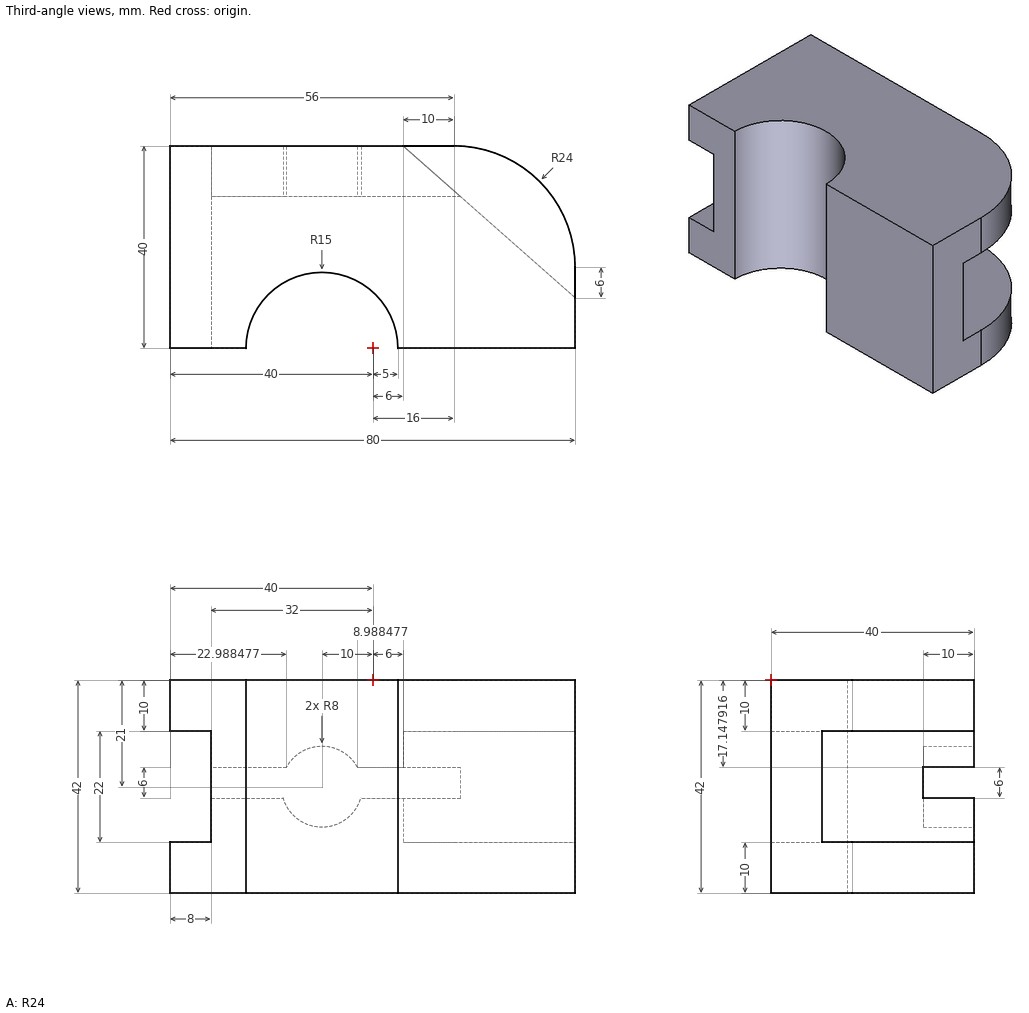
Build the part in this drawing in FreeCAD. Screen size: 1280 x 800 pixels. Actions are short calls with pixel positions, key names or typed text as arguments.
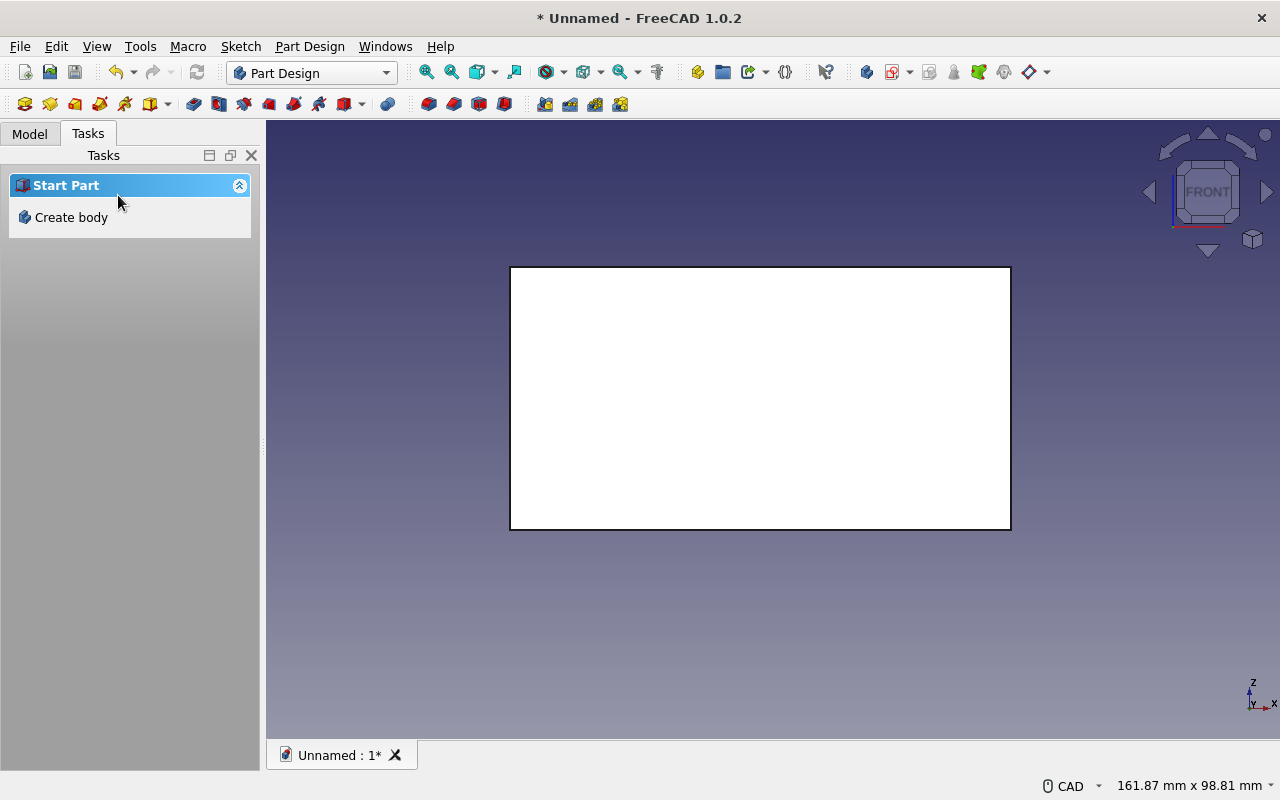
key(3)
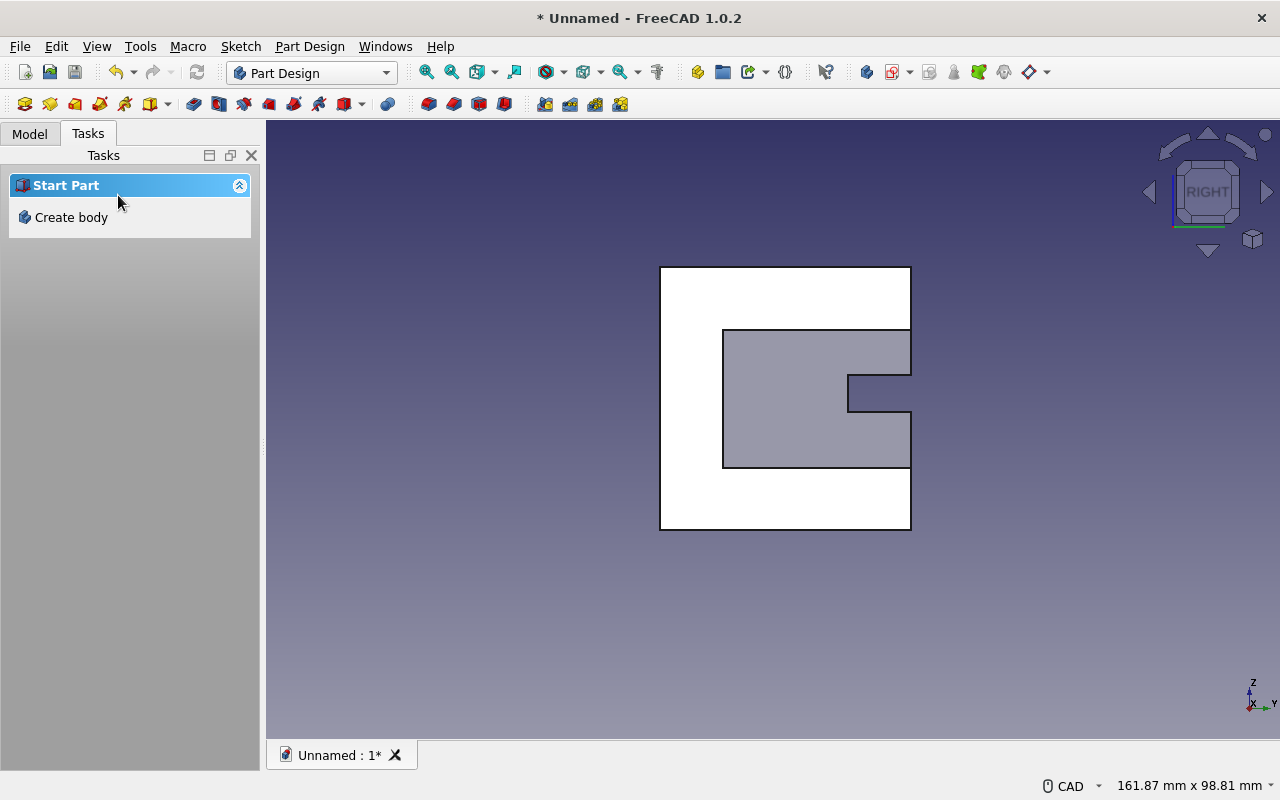
key(v)
key(f)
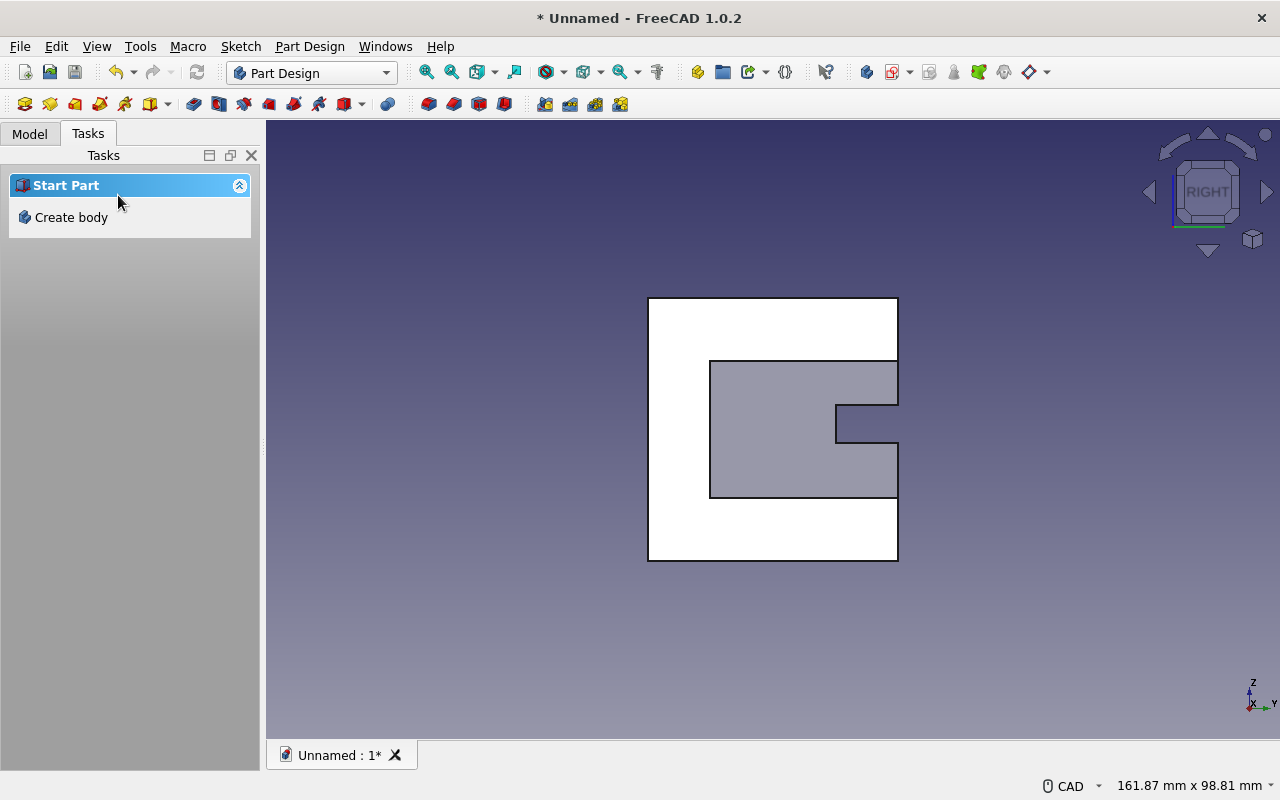
click(898, 529)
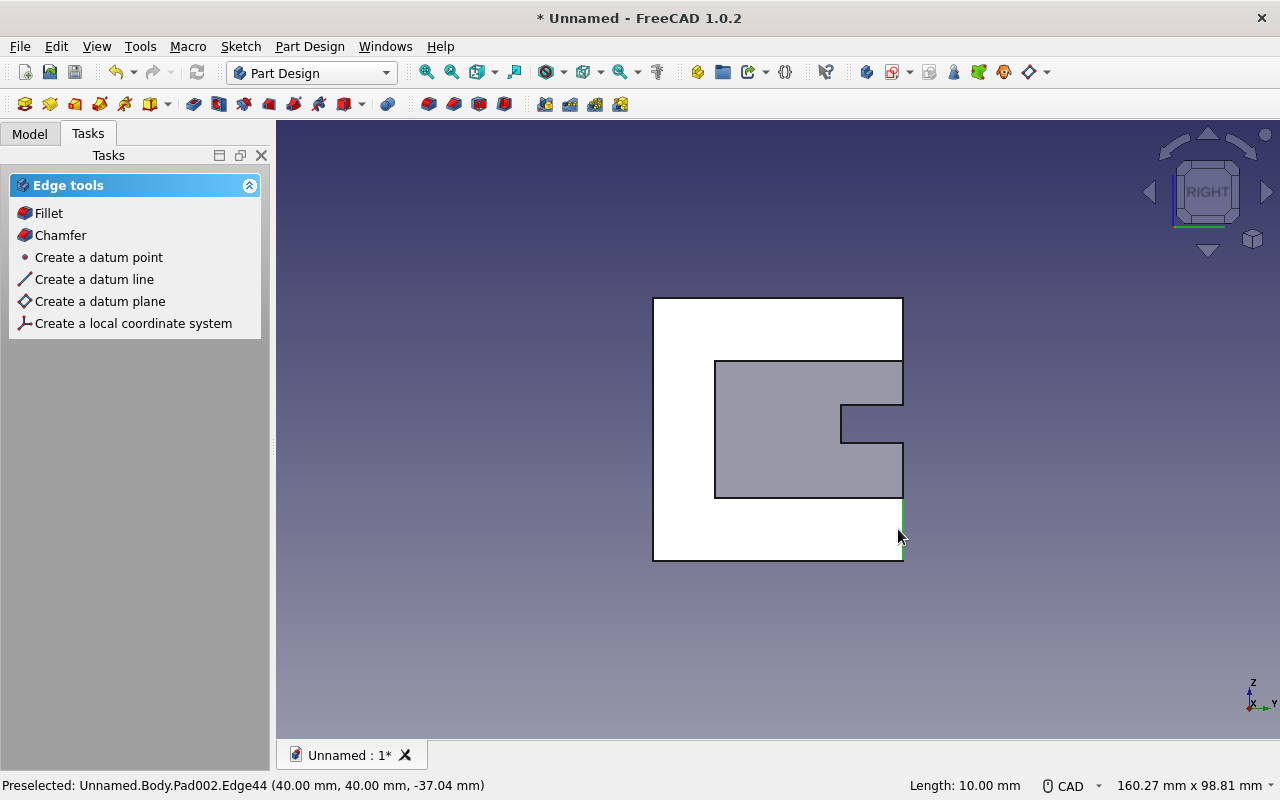
click(903, 328, ctrl)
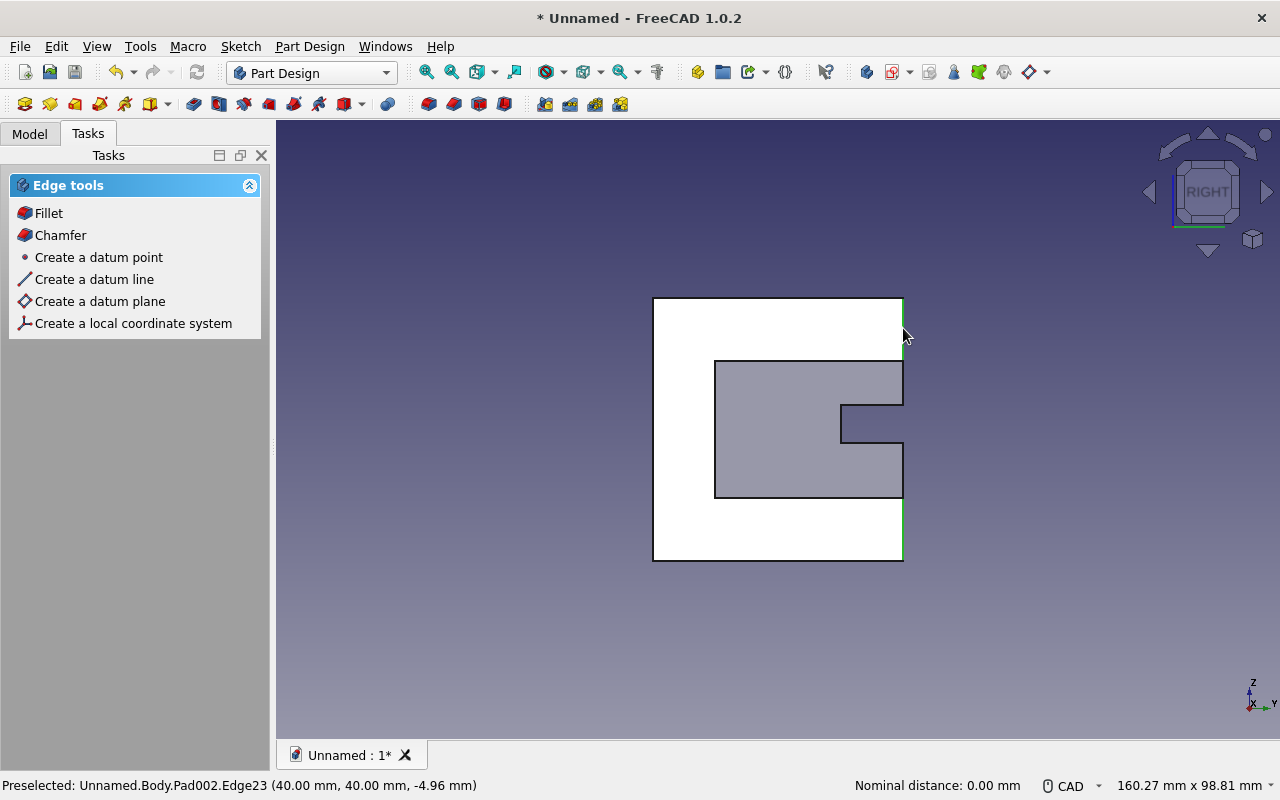
click(429, 104)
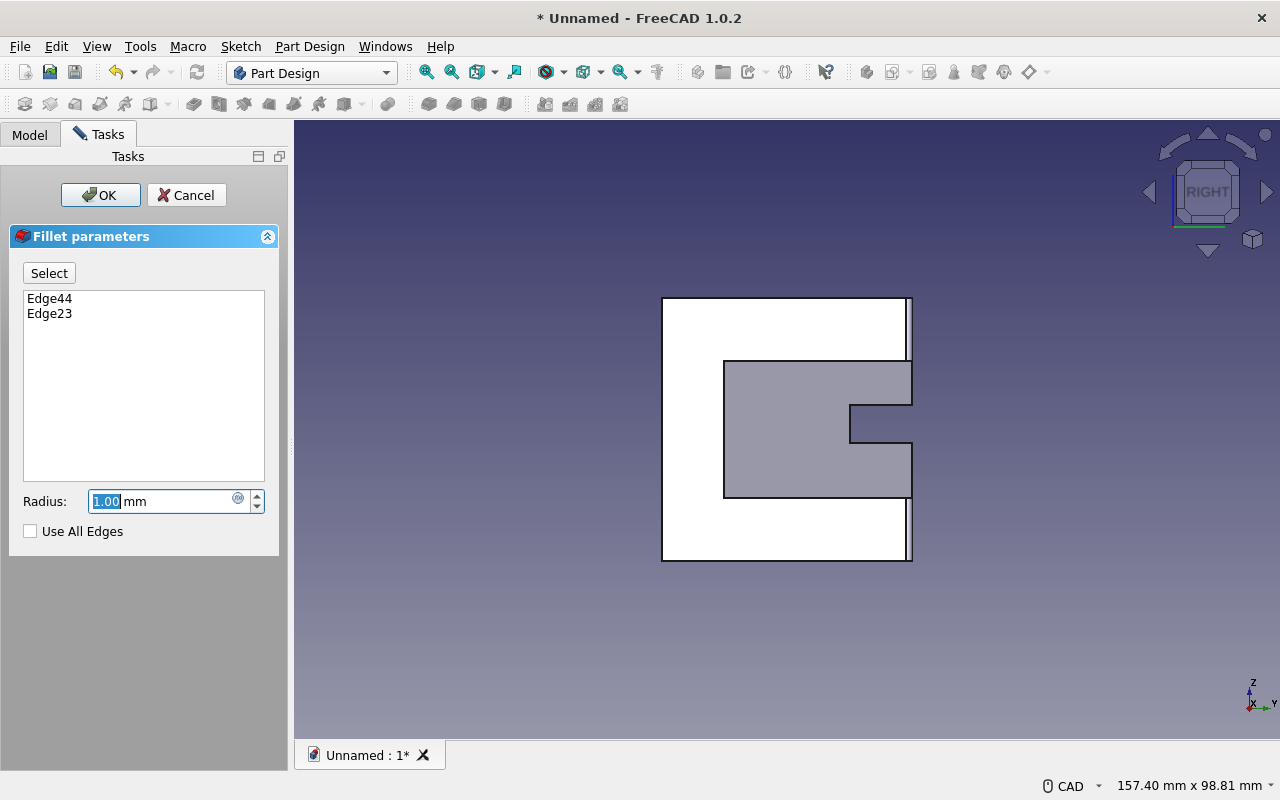
text(24)
key(Tab)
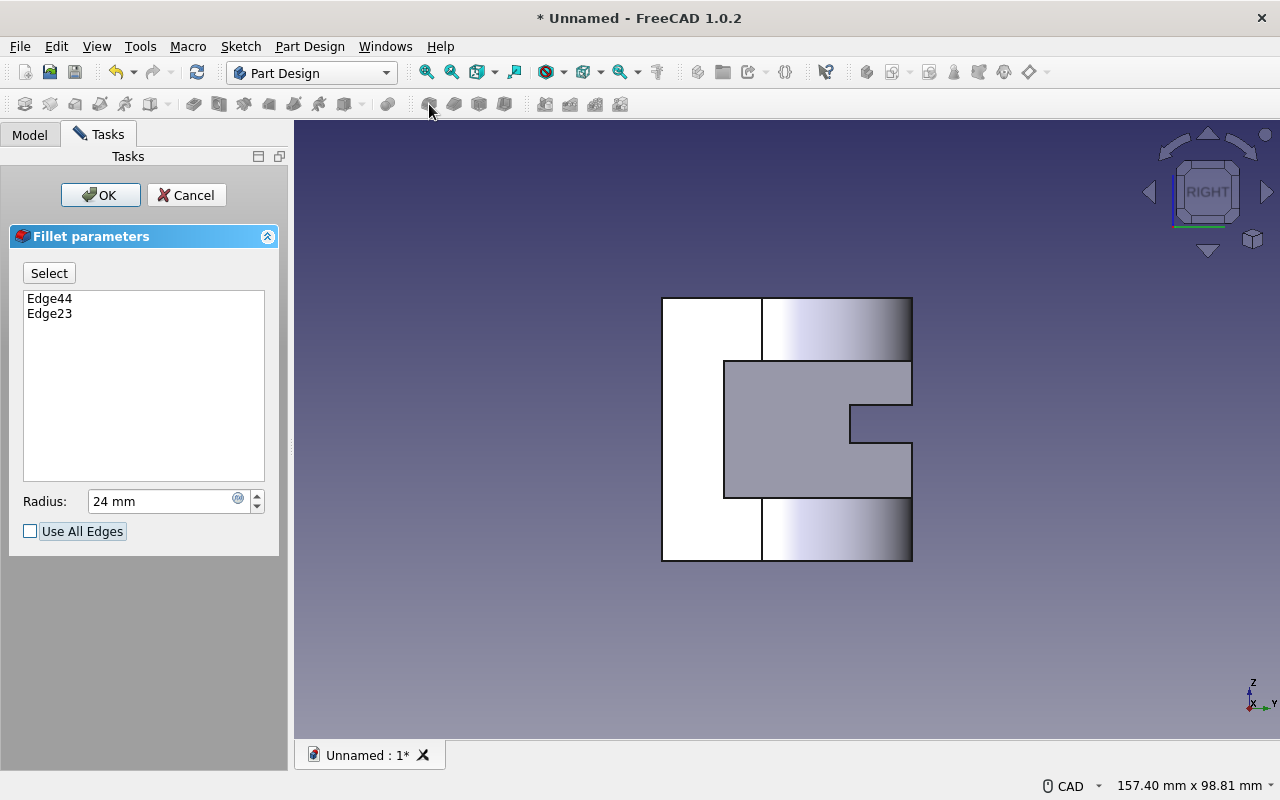
click(101, 195)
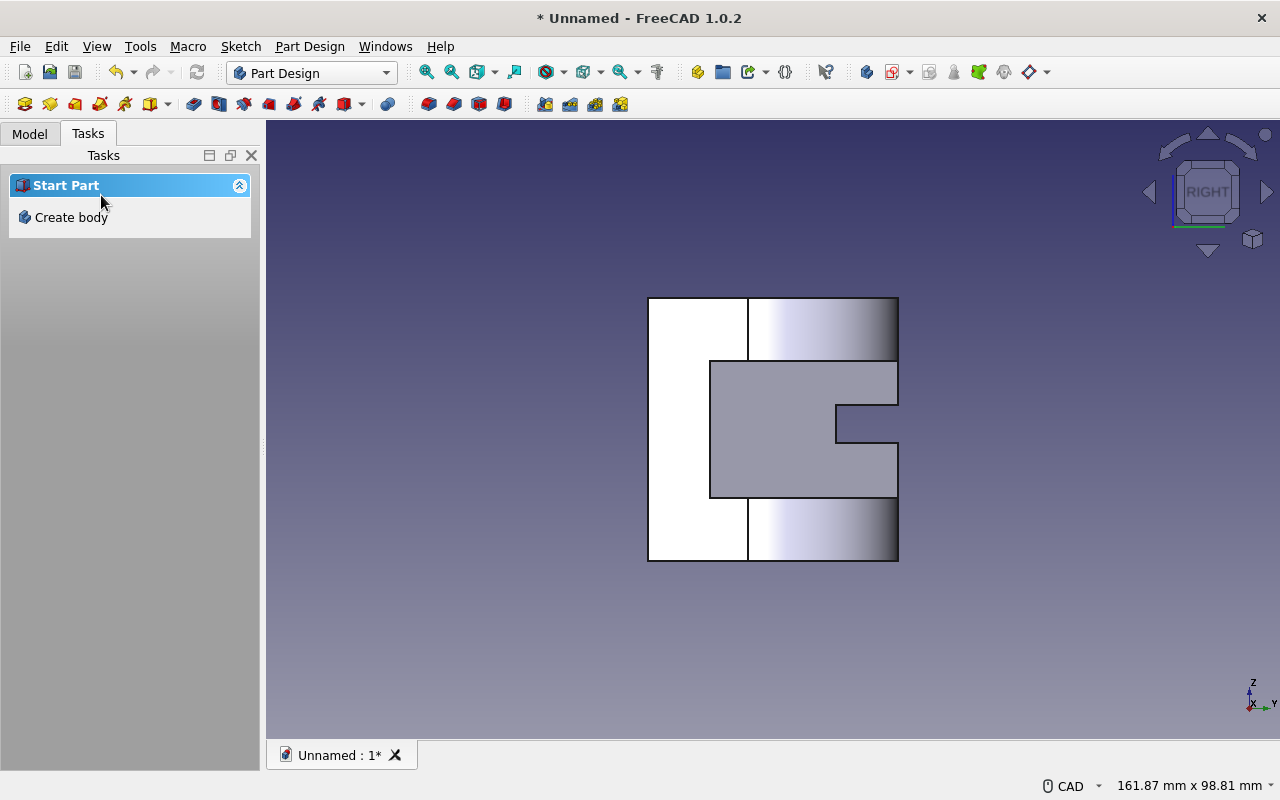
key(v)
key(f)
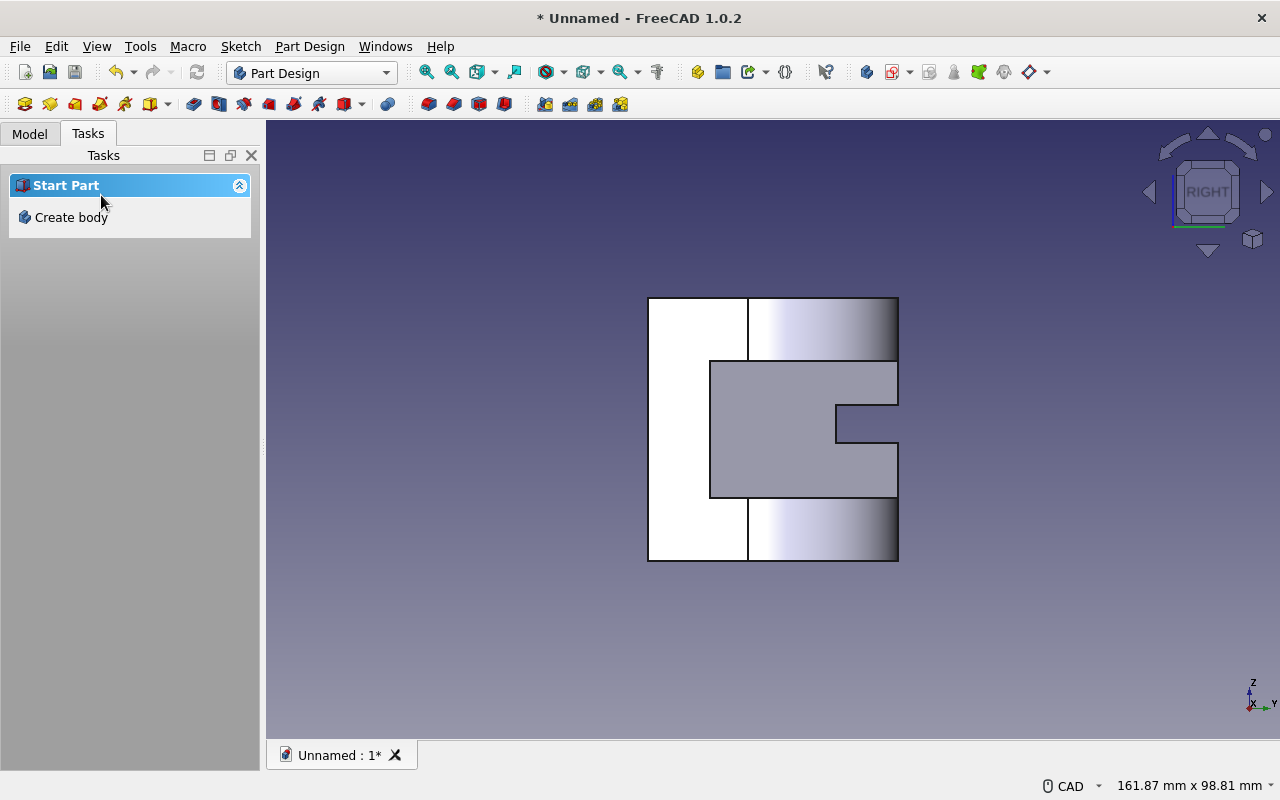
click(892, 72)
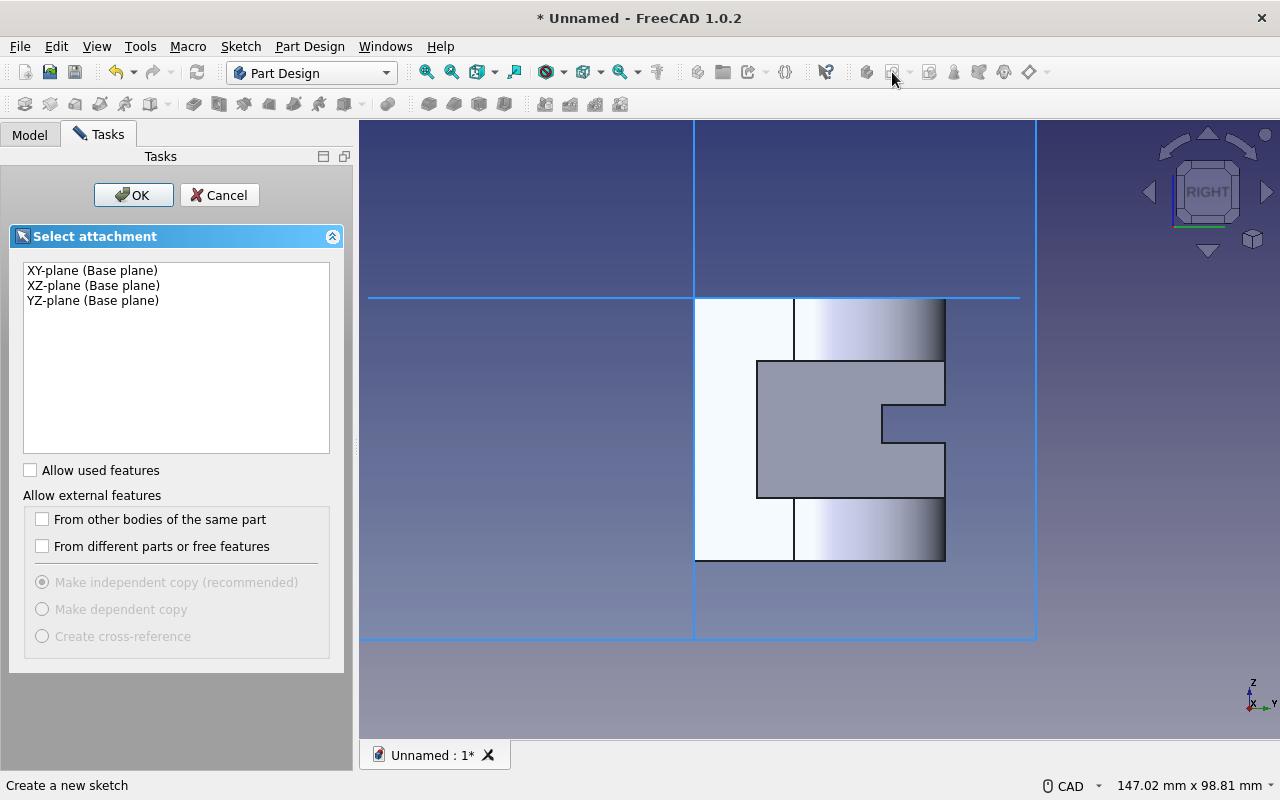
click(84, 270)